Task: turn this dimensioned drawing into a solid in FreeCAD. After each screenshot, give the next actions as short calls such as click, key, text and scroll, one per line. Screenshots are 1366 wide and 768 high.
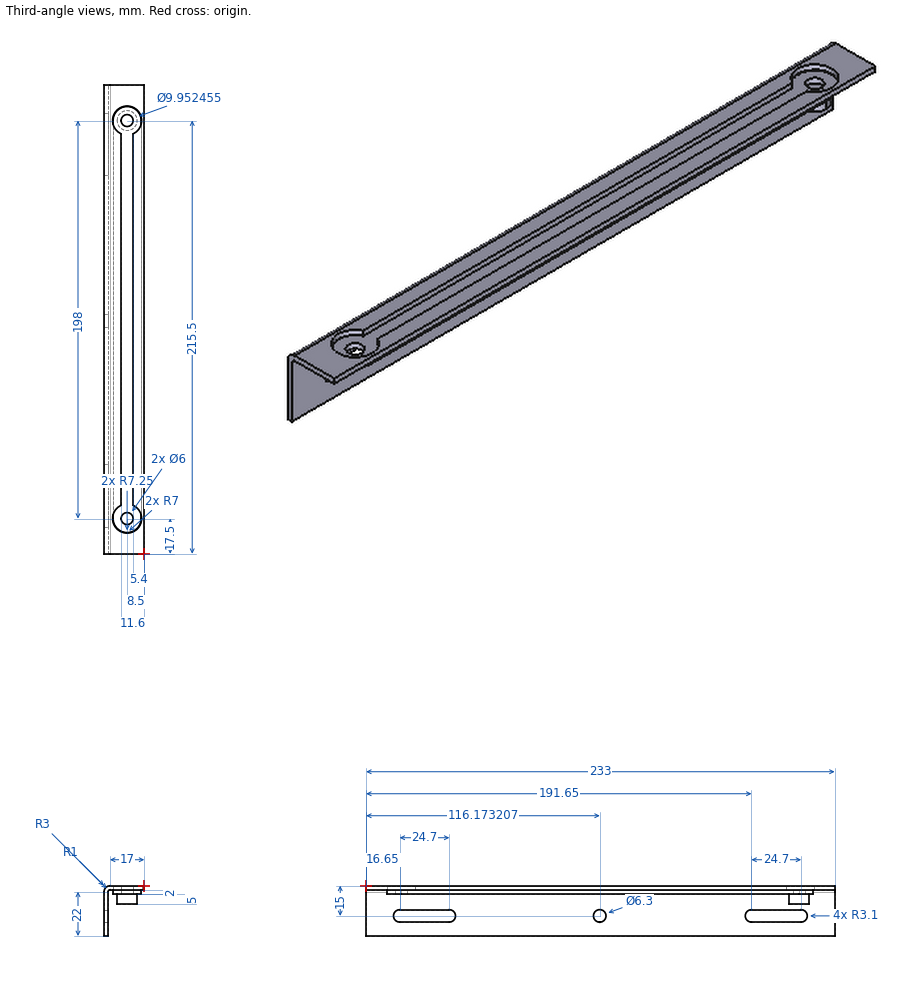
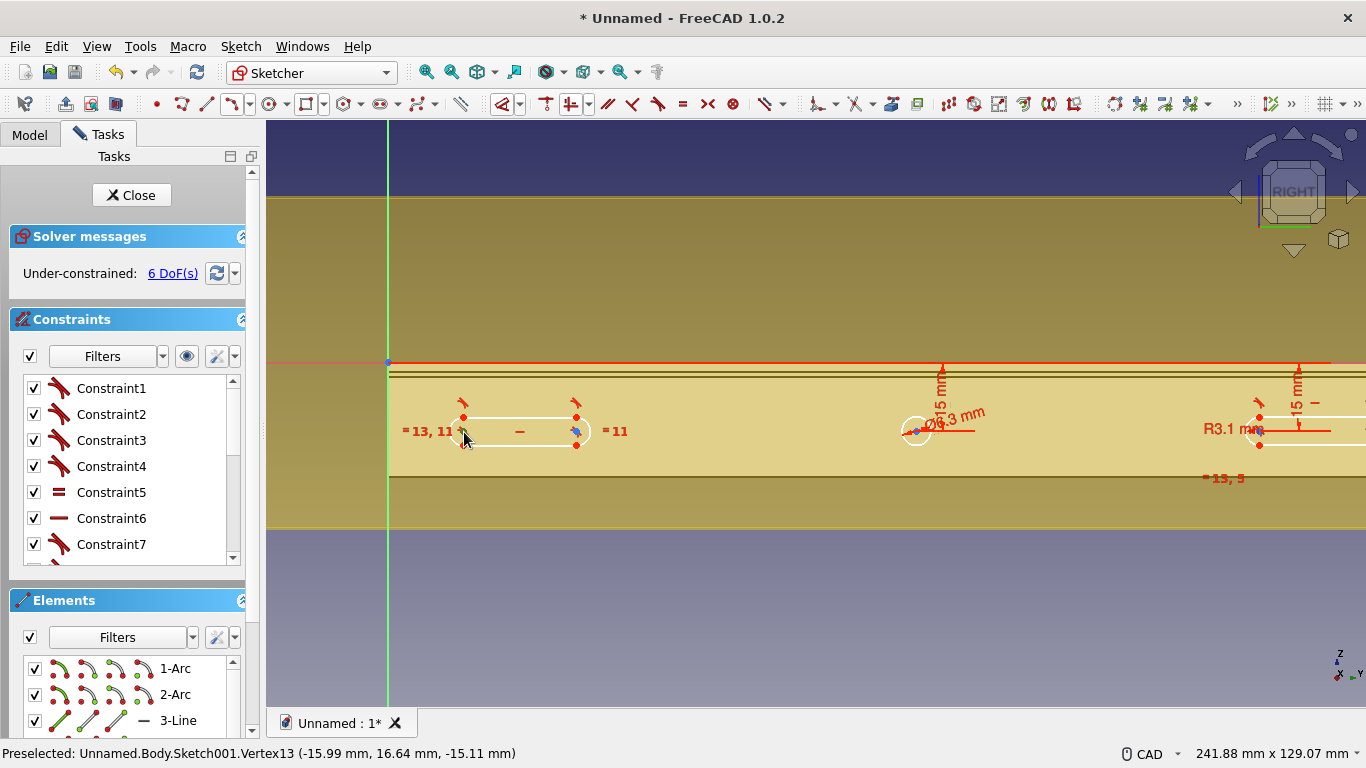
click(520, 104)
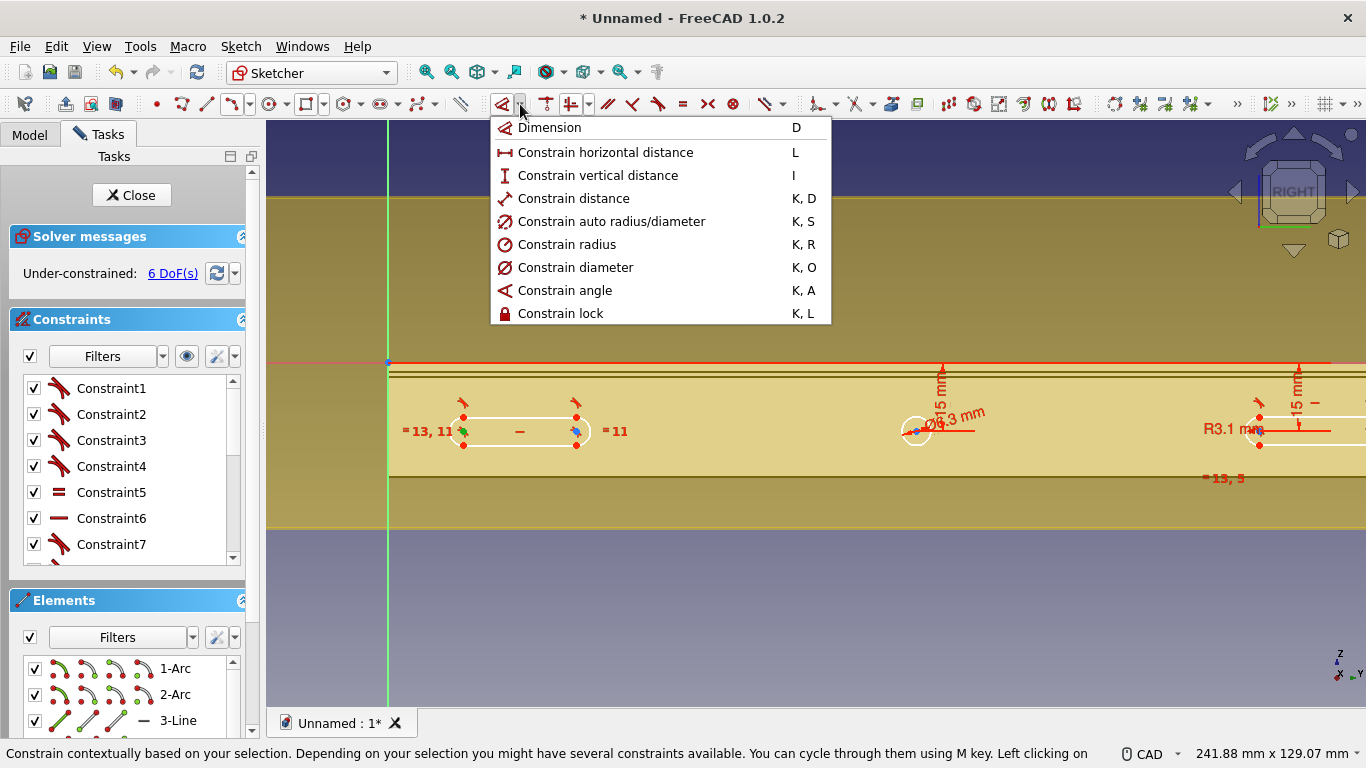
click(661, 176)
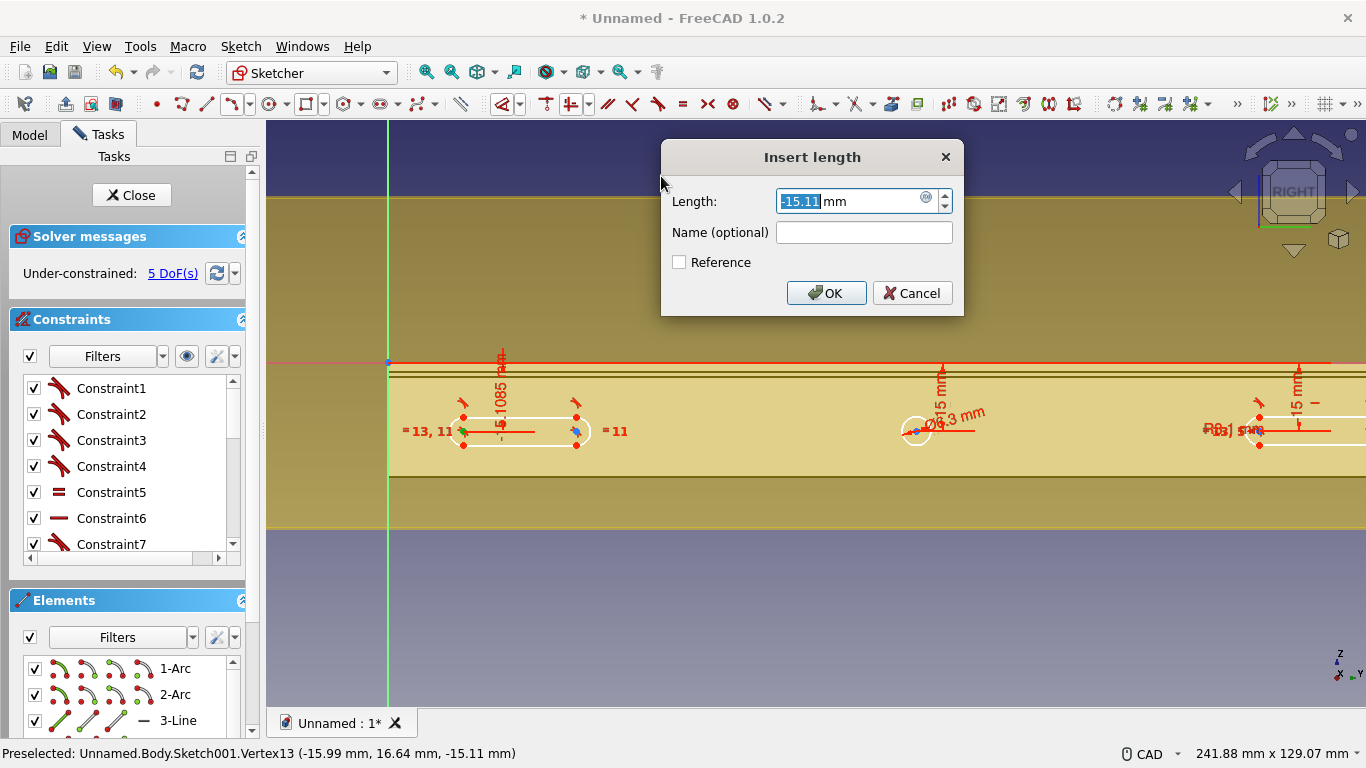
text(-15)
key(Return)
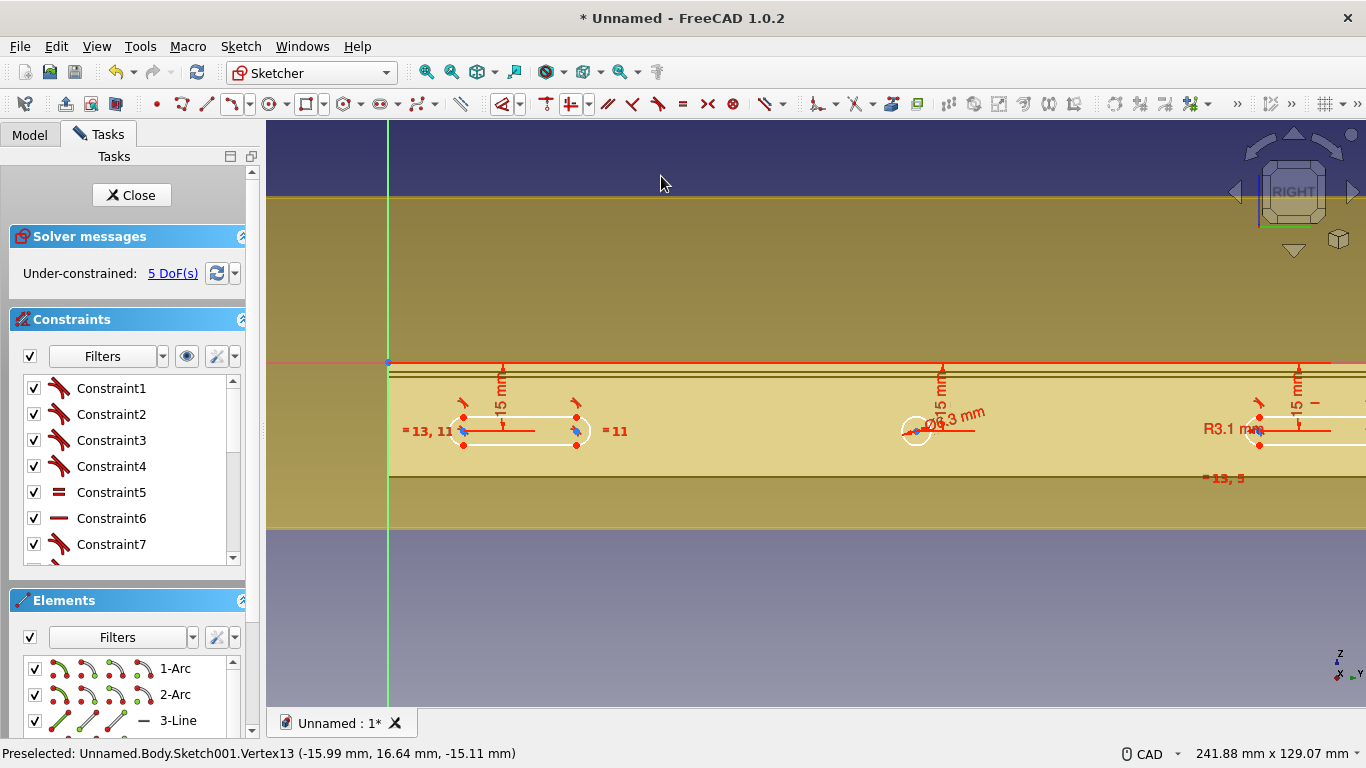
scroll(464, 432, down, 2)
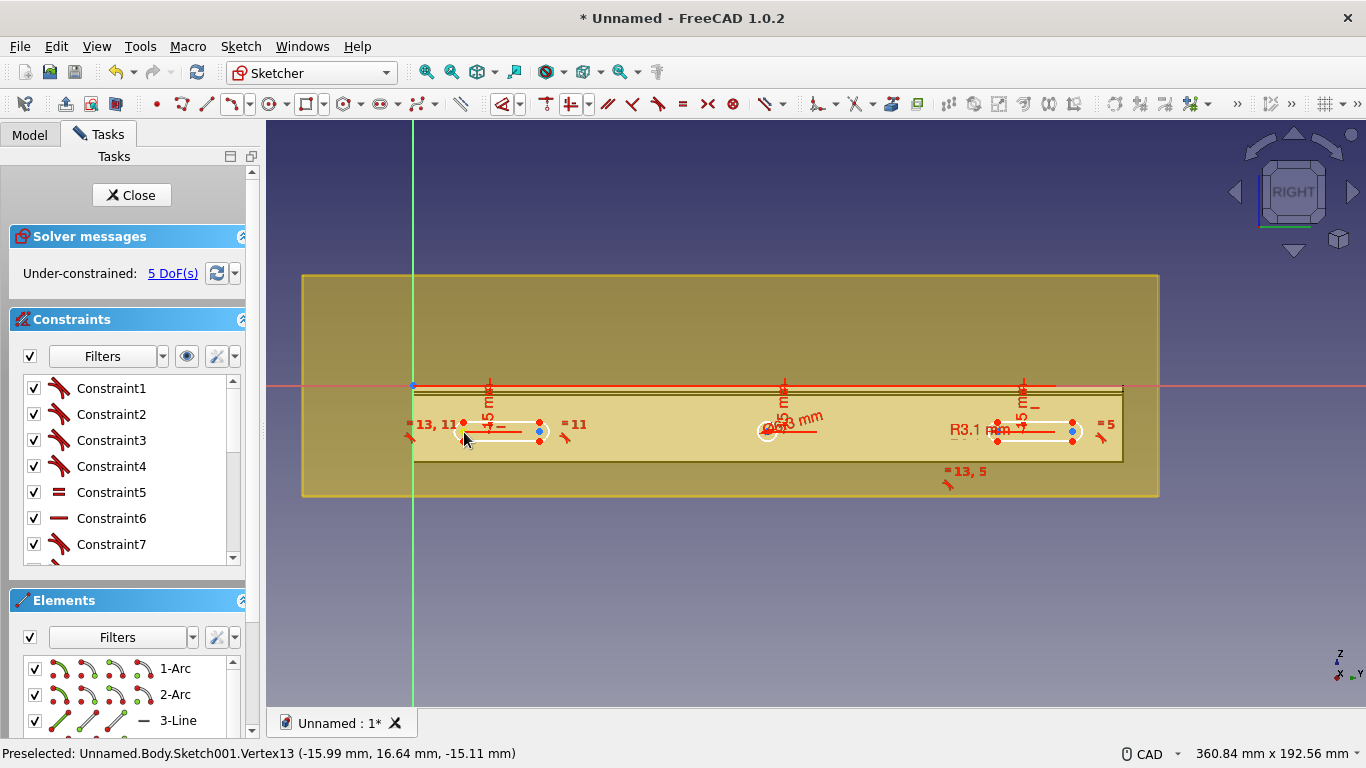
click(1050, 422)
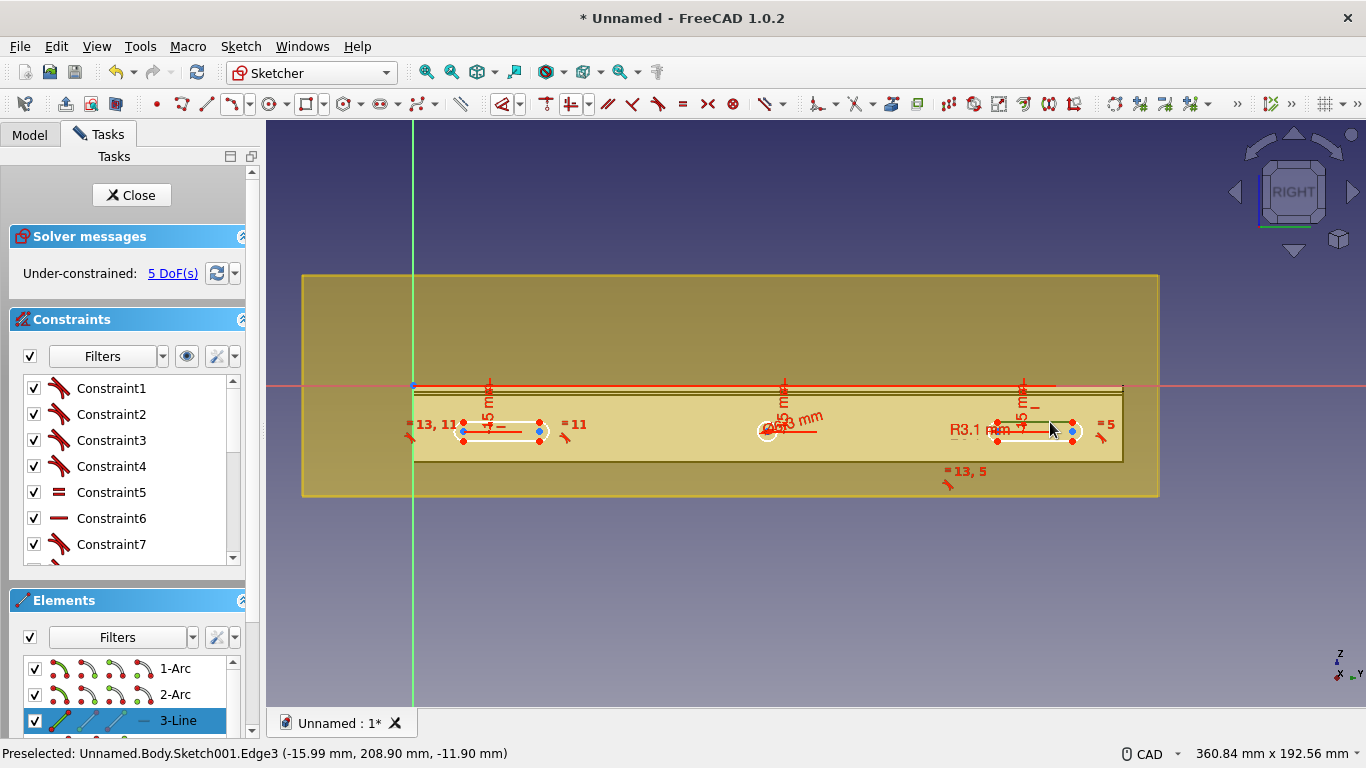
key(l)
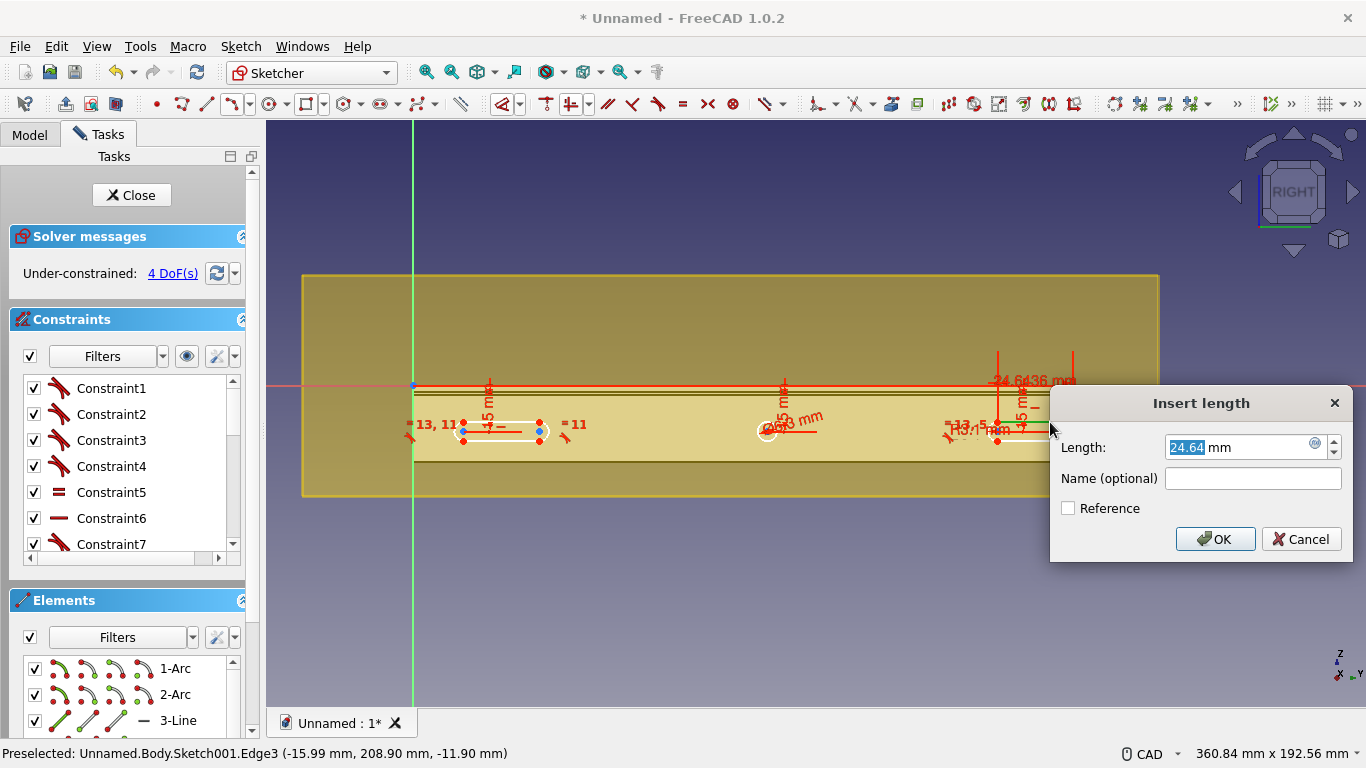
text(24.7)
key(Return)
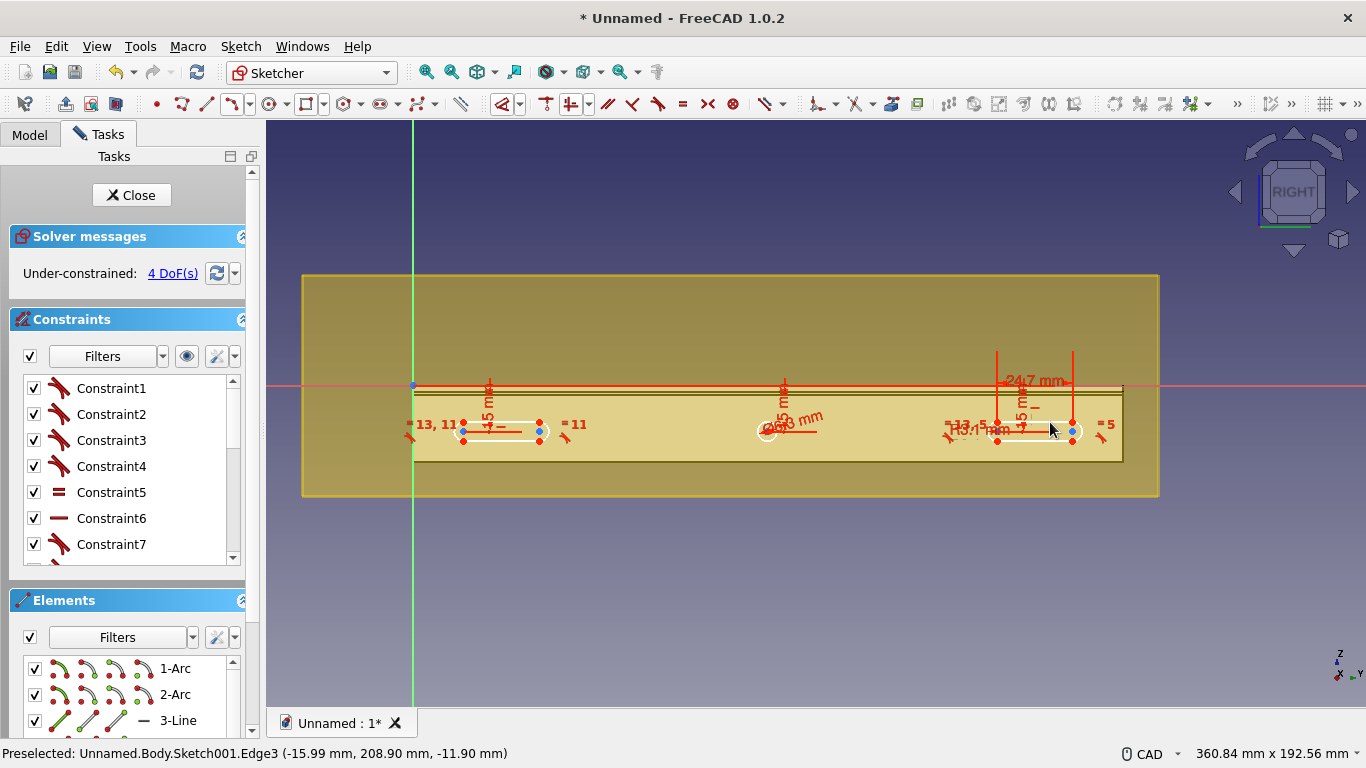
click(517, 422)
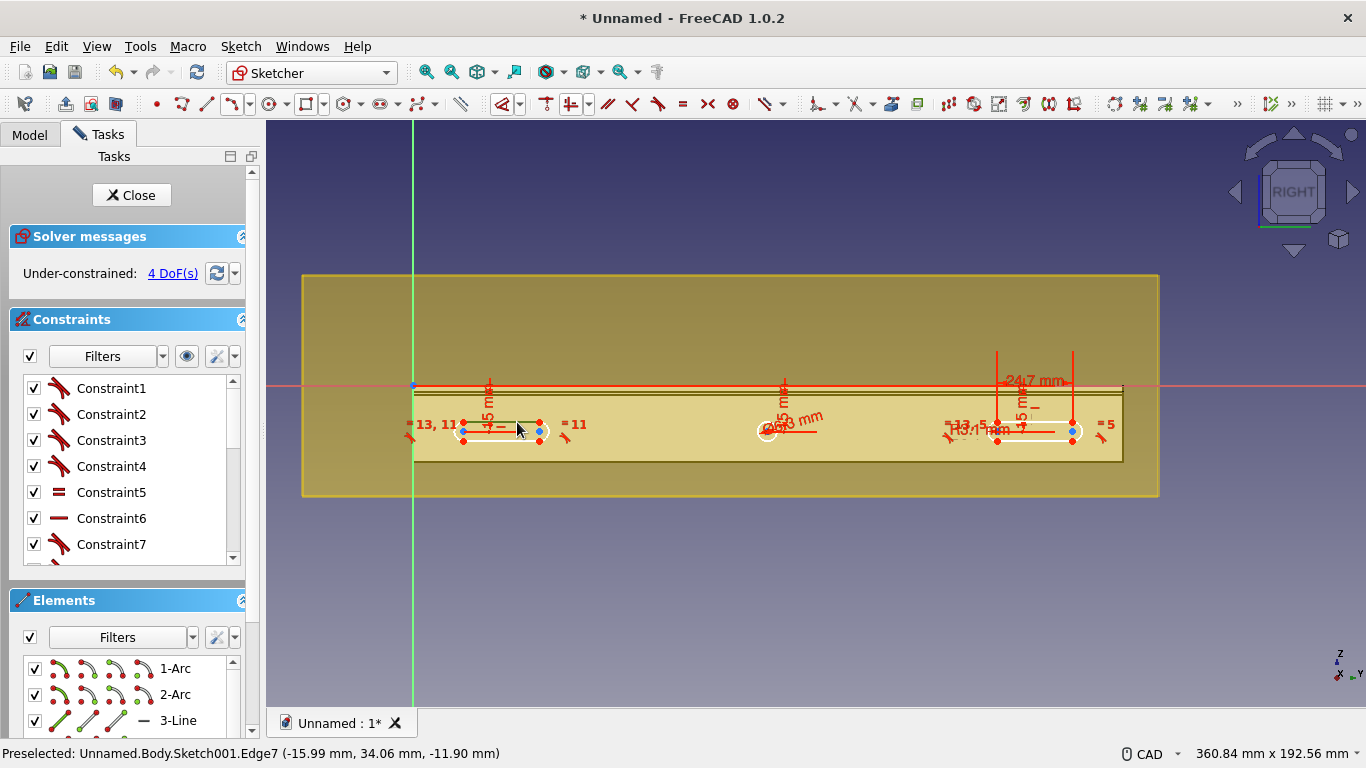
click(520, 104)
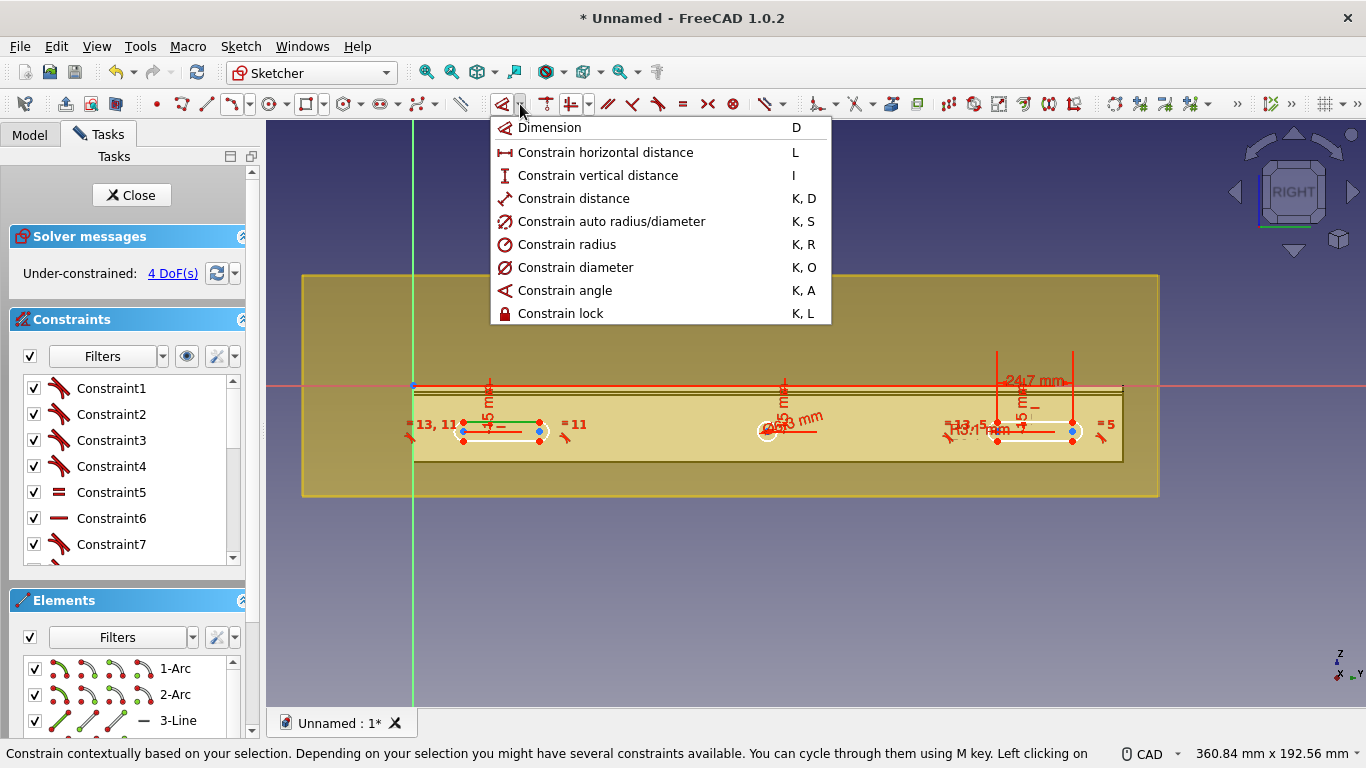
click(661, 152)